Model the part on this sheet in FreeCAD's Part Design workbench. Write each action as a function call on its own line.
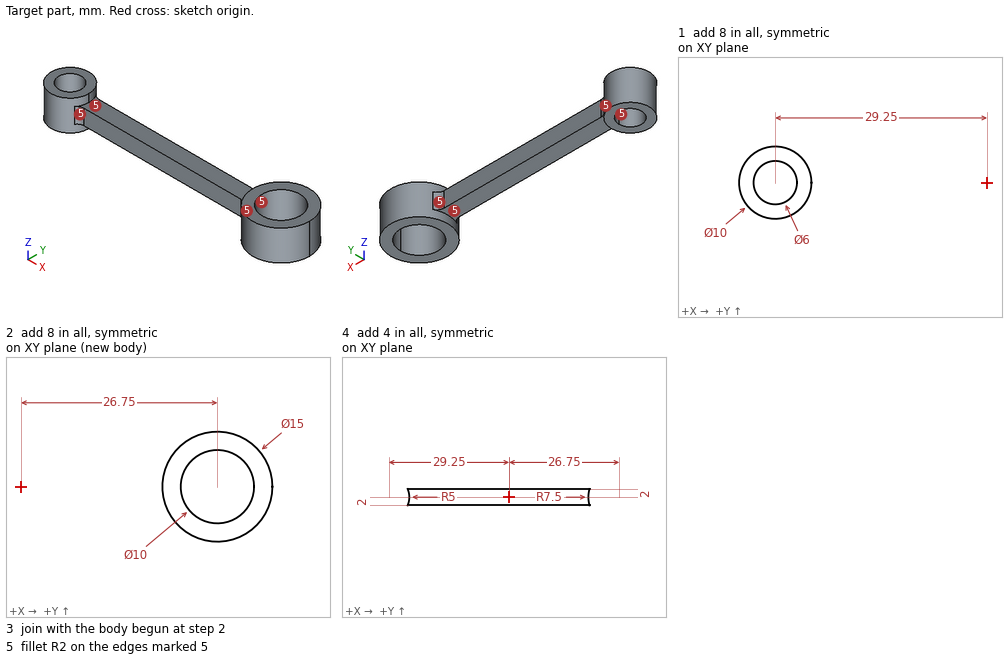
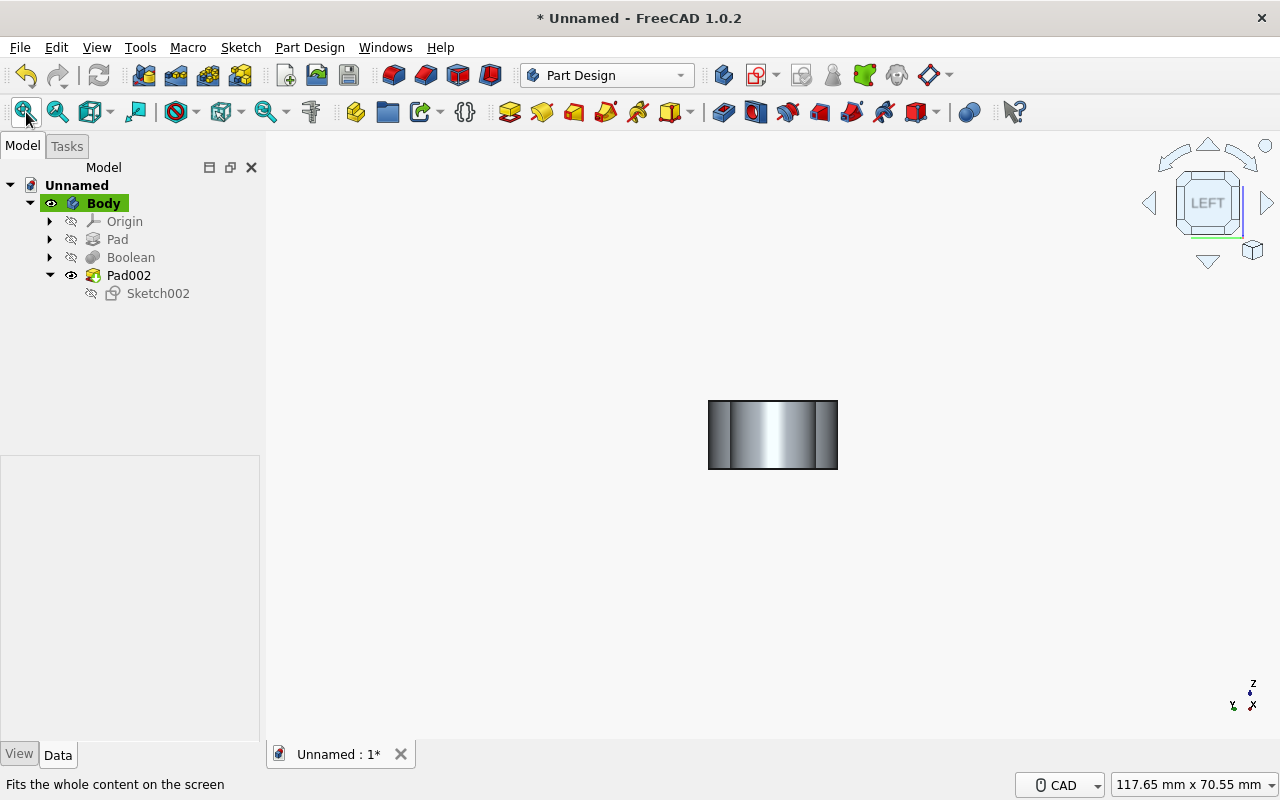
key(v)
key(3)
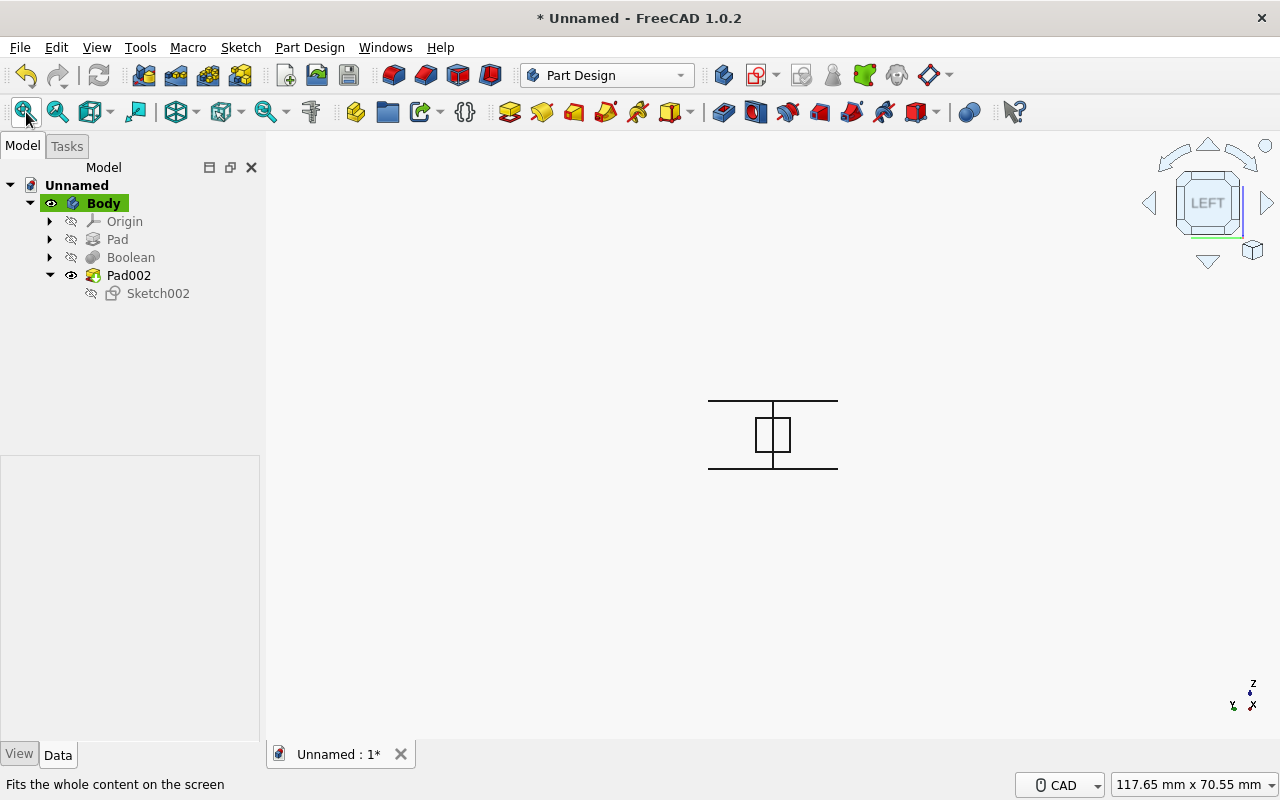
key(0)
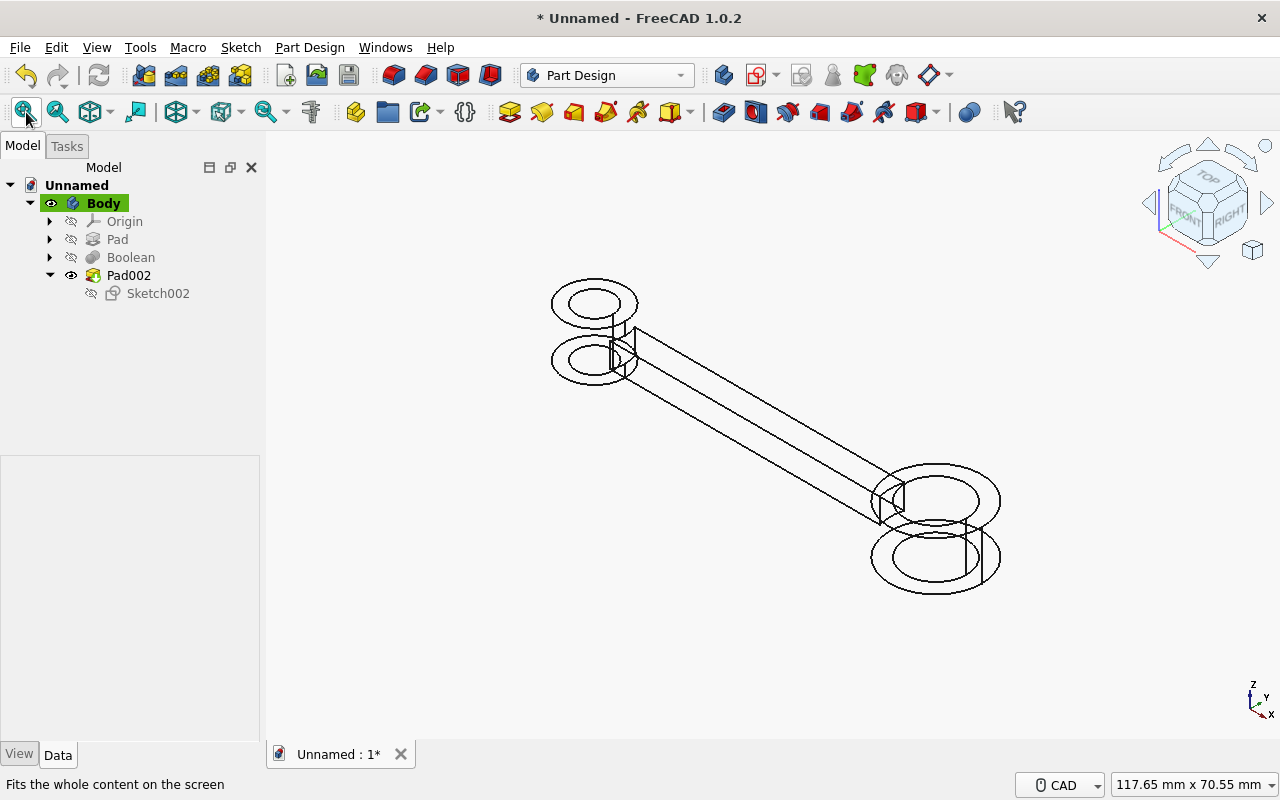
click(880, 507)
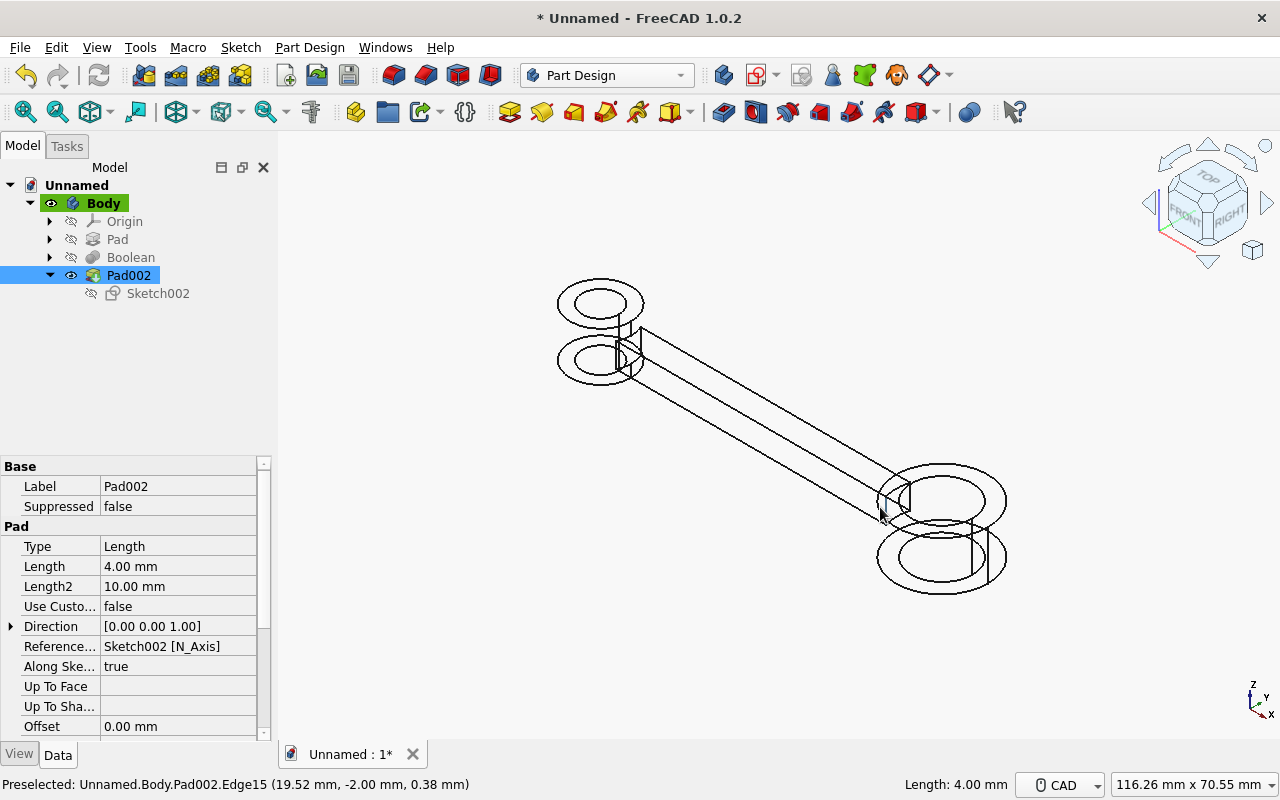
click(910, 496, ctrl)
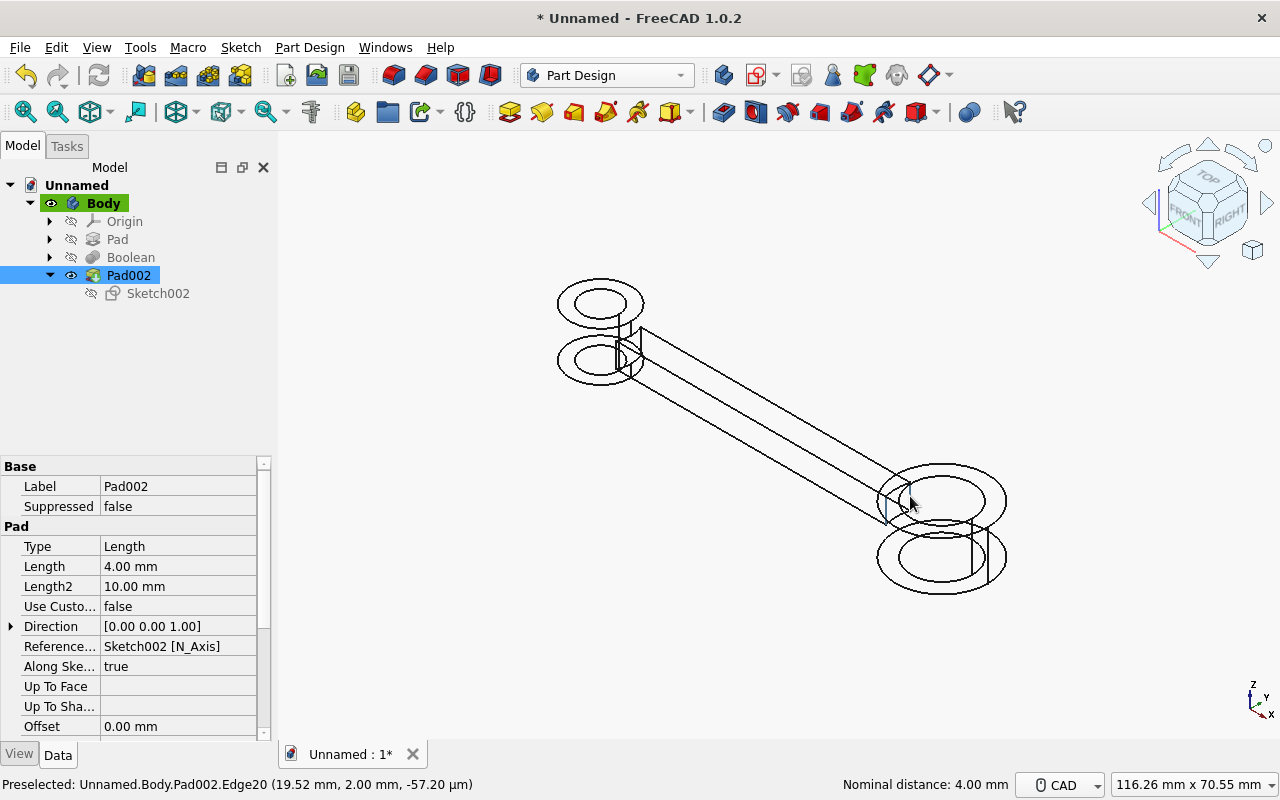
click(641, 340, ctrl)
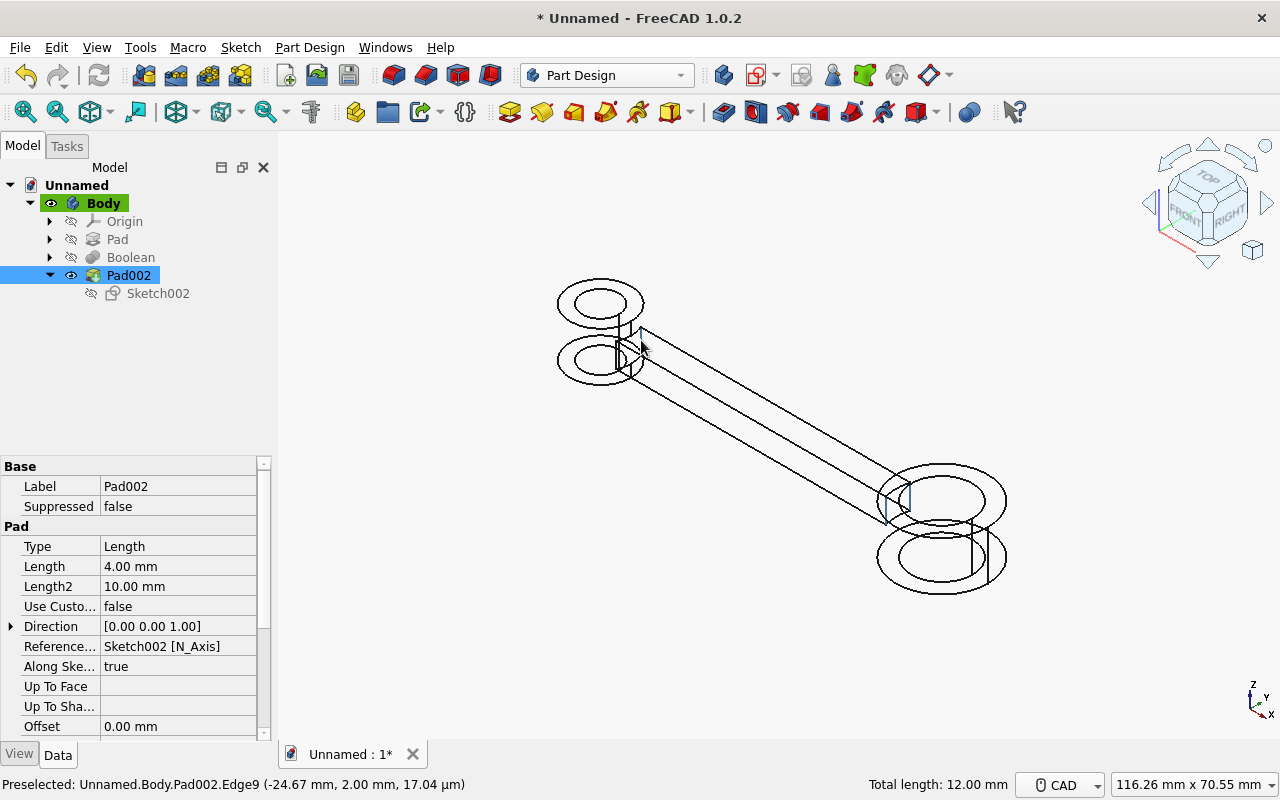
click(616, 354, ctrl)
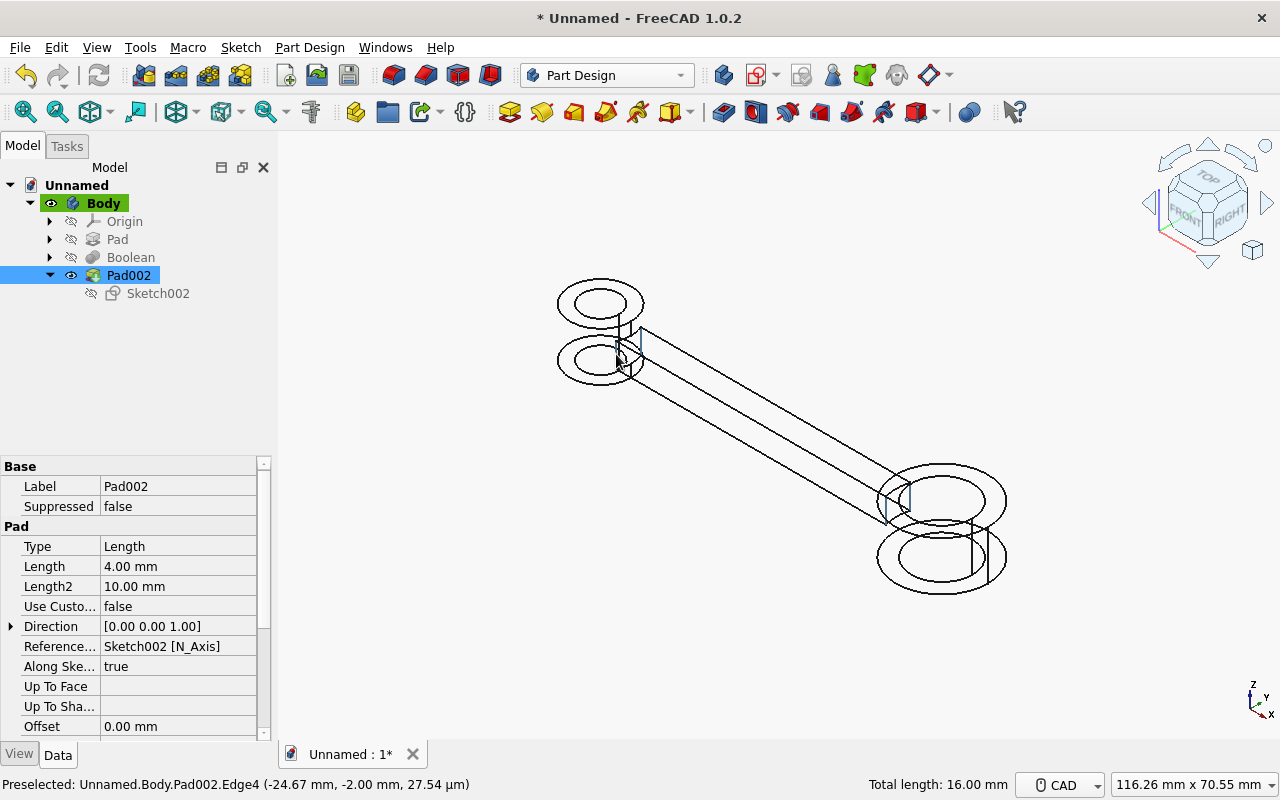
key(v)
key(1)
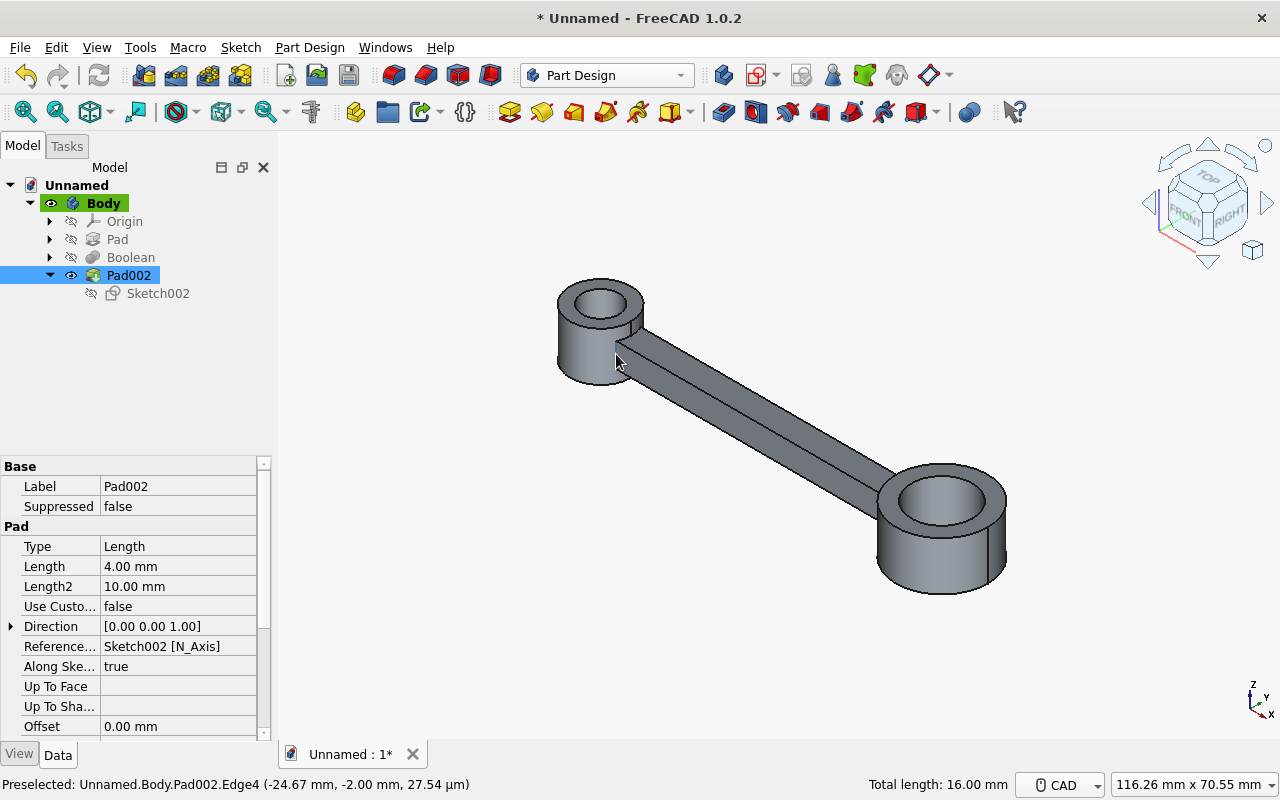
click(394, 76)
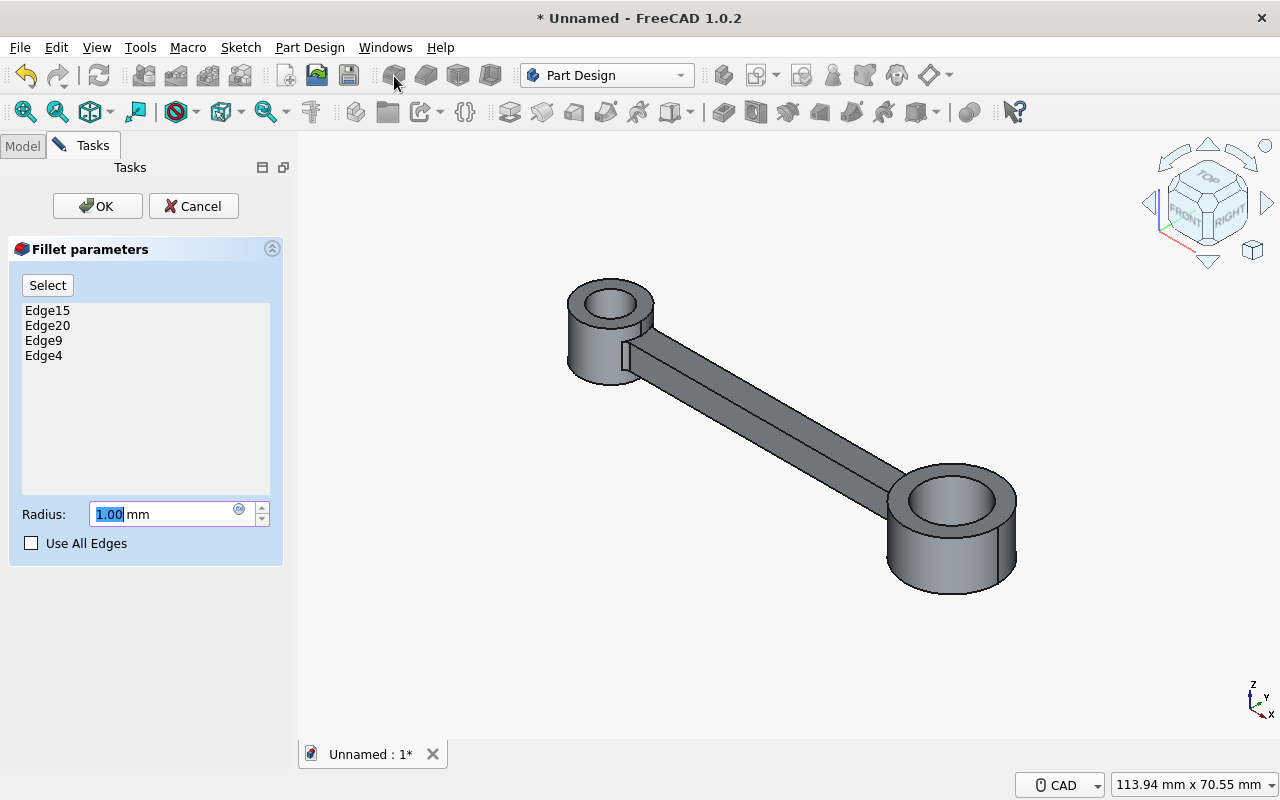
text(2)
key(Tab)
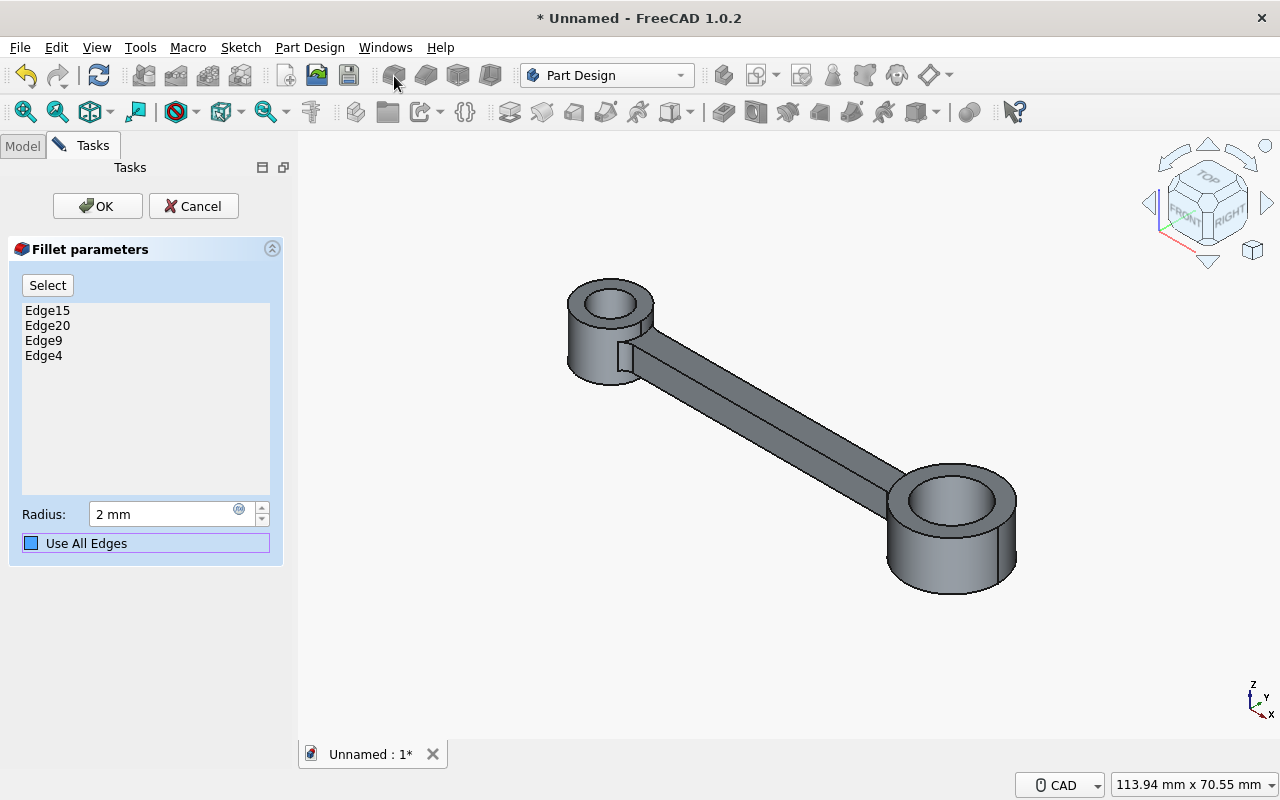
click(98, 206)